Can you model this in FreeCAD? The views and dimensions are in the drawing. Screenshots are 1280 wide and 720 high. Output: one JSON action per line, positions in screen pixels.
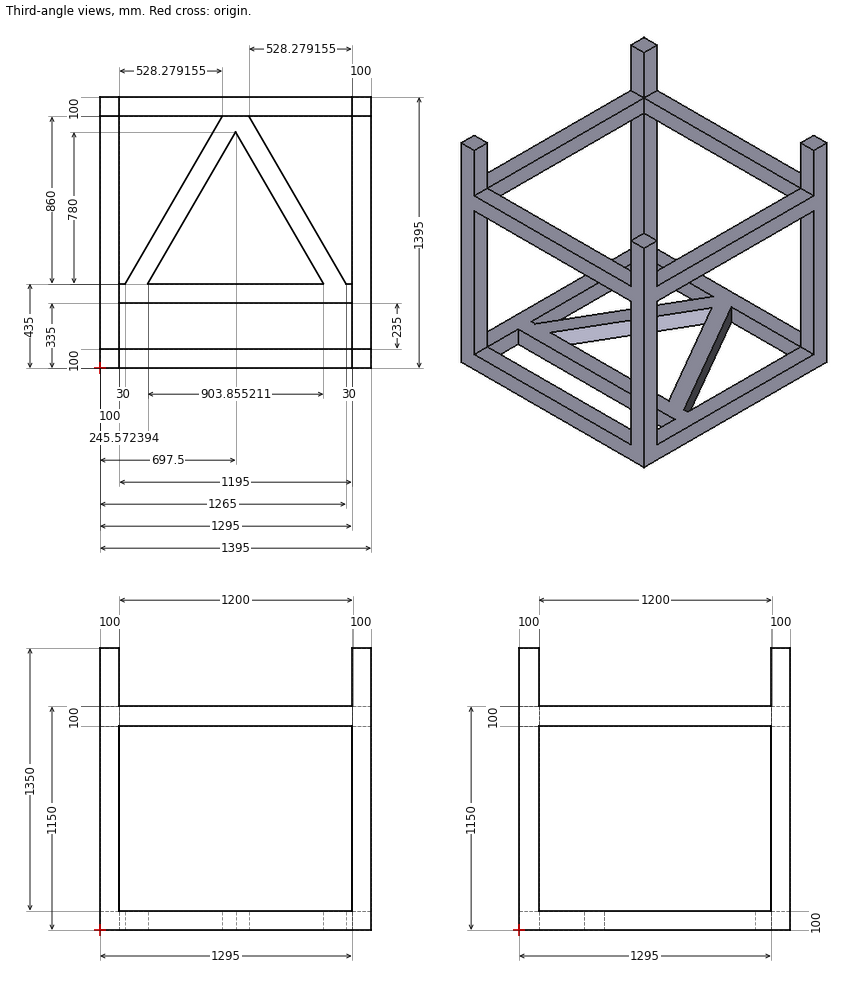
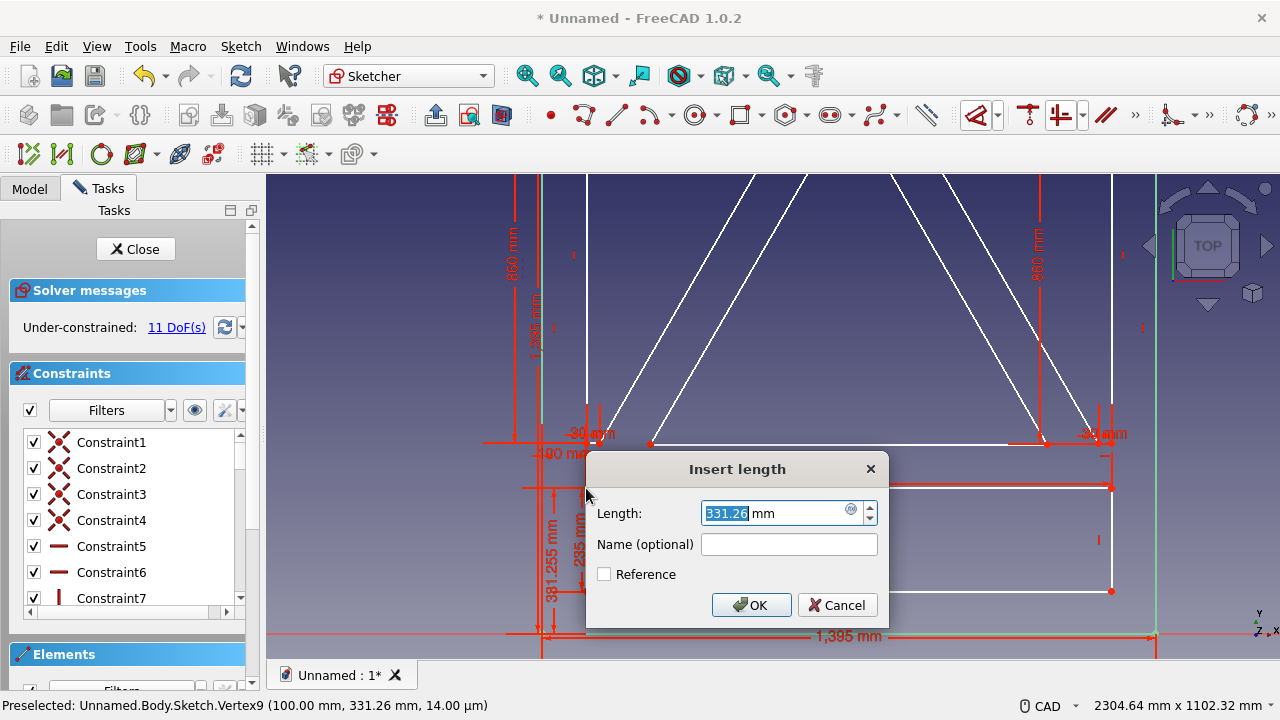
{"action": "type", "text": "335"}
{"action": "key", "text": "Return"}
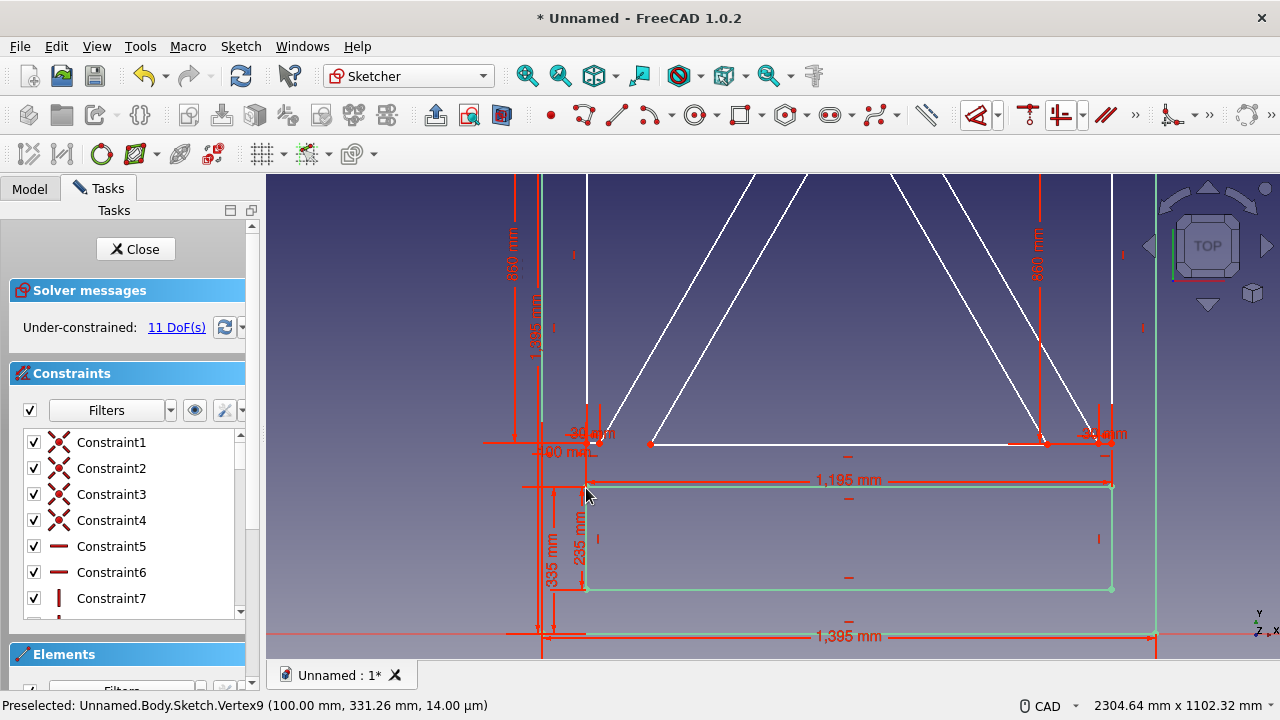
{"action": "left_click", "coordinate": [587, 443]}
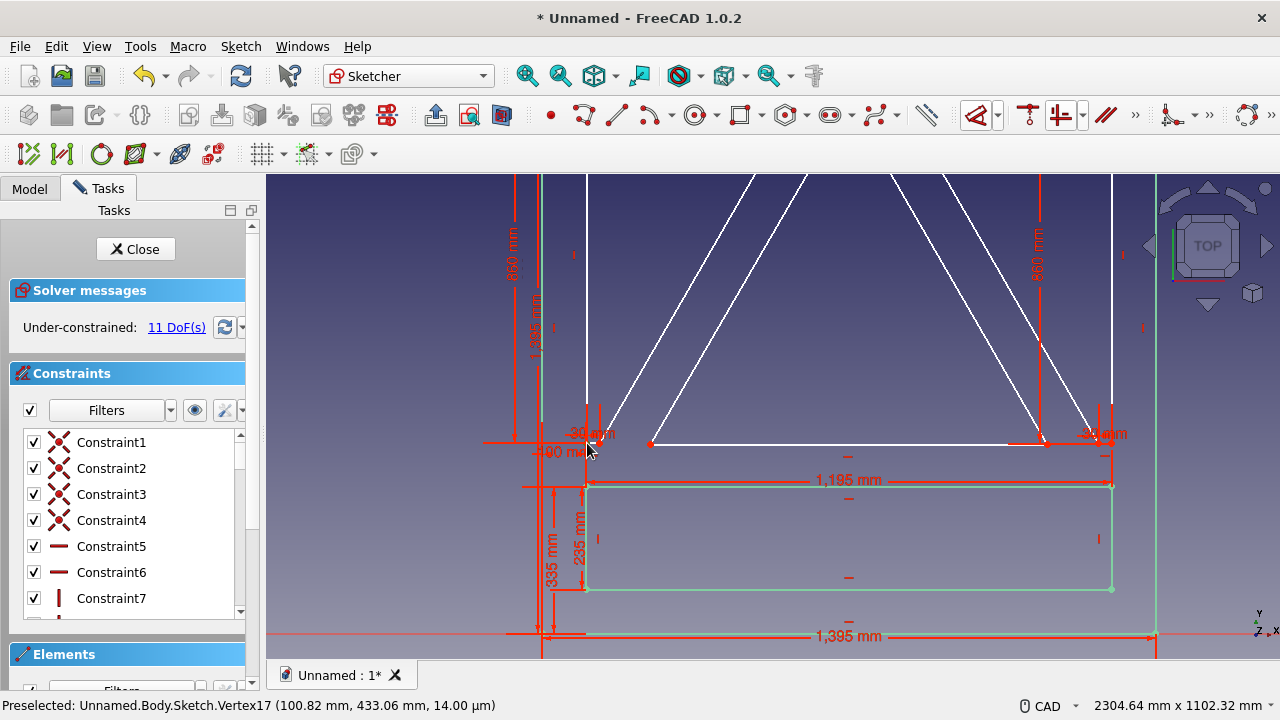
{"action": "left_click", "coordinate": [998, 116]}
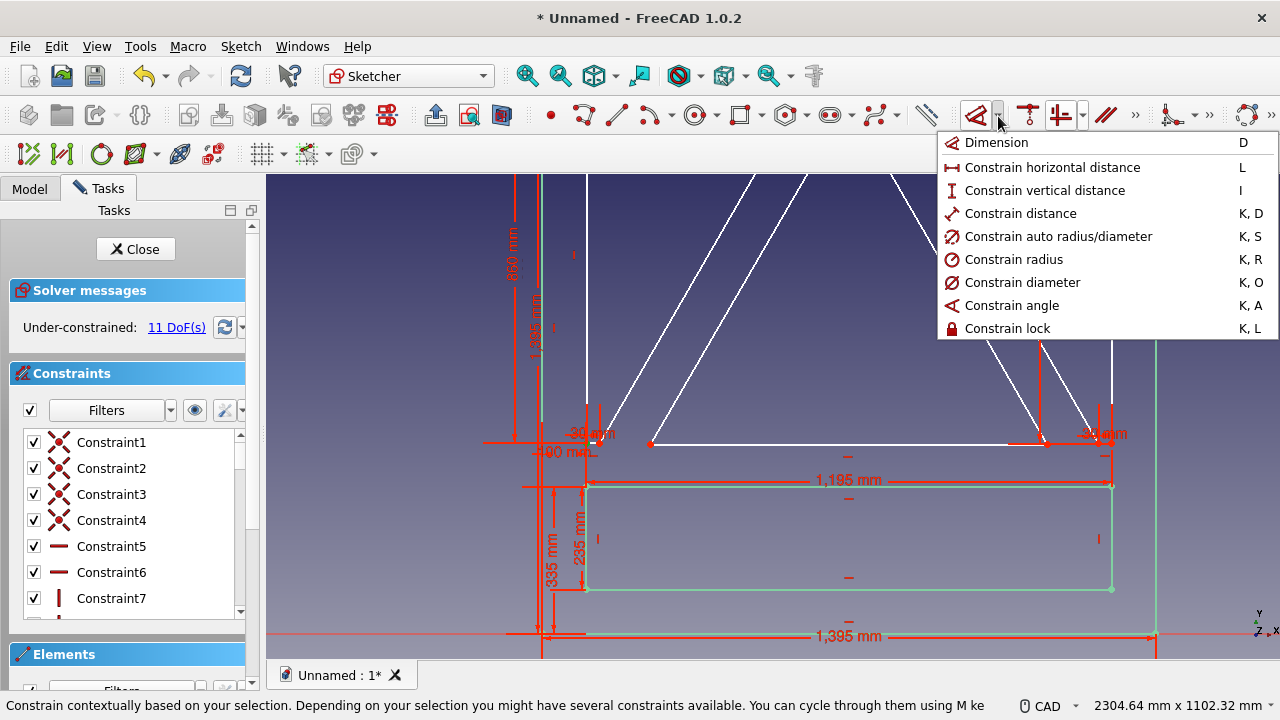
{"action": "left_click", "coordinate": [1108, 168]}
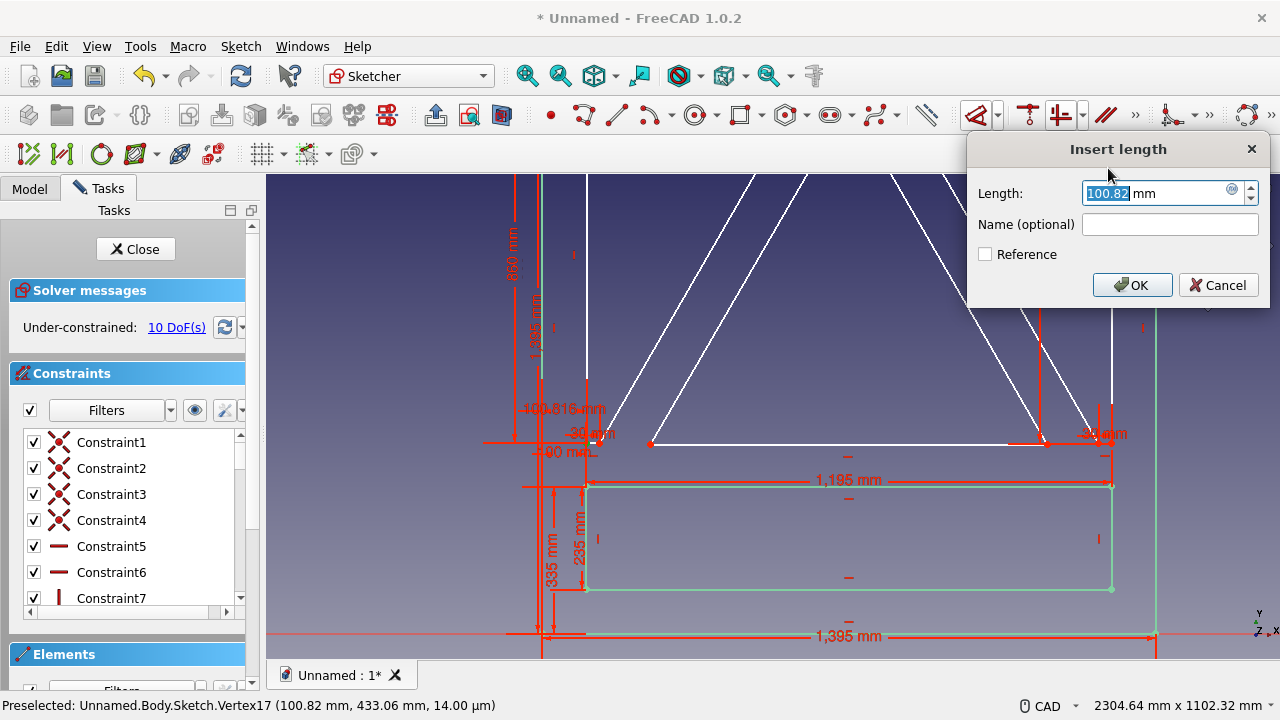
{"action": "type", "text": "100"}
{"action": "key", "text": "Return"}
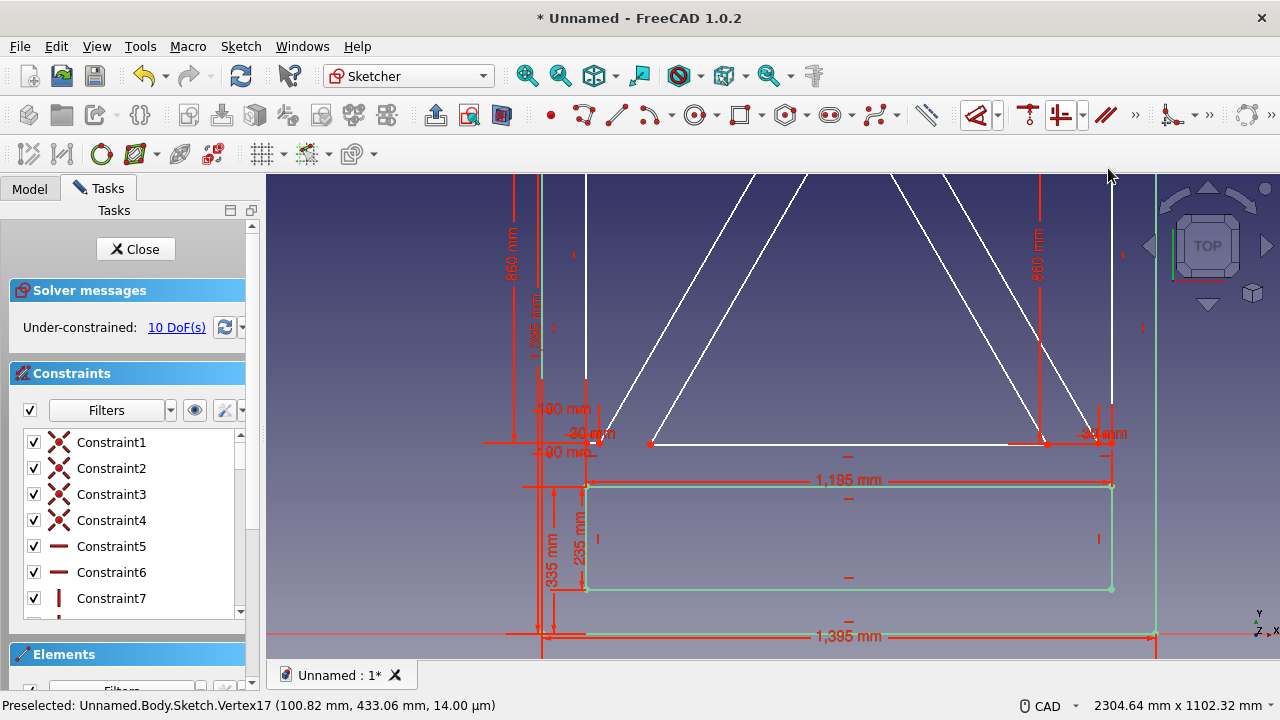
{"action": "left_click", "coordinate": [586, 443]}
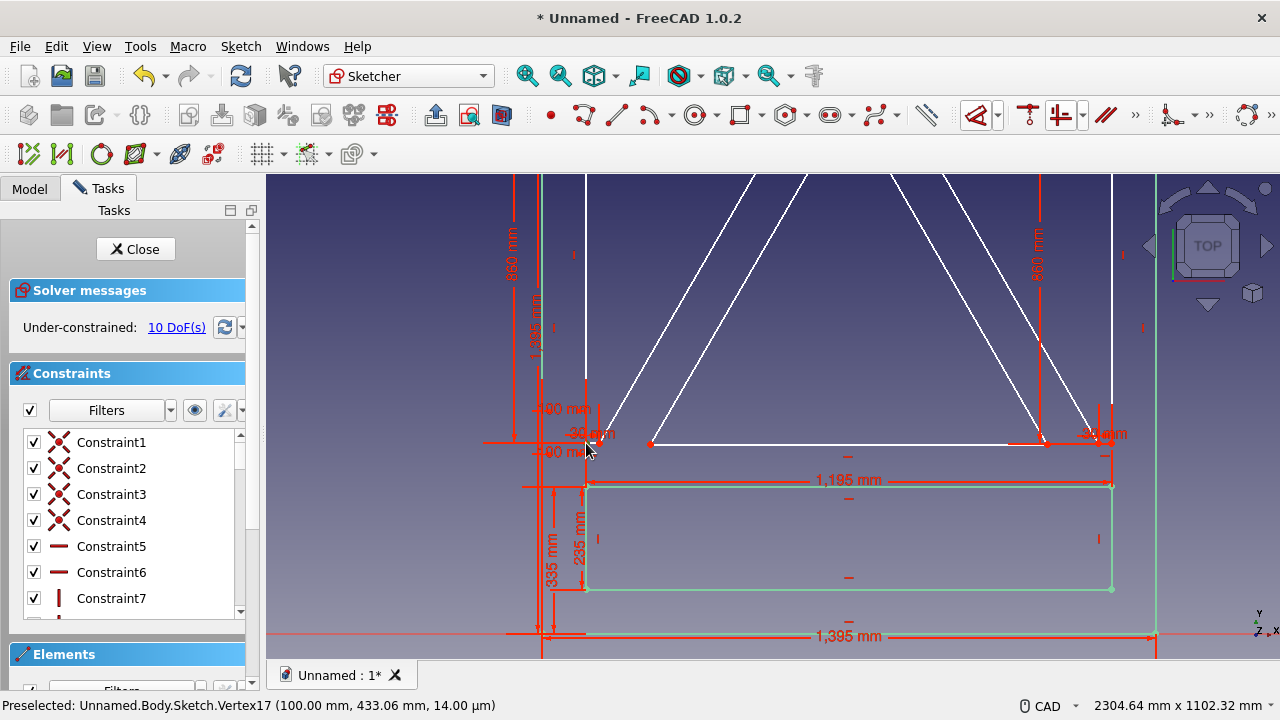
{"action": "key", "text": "i"}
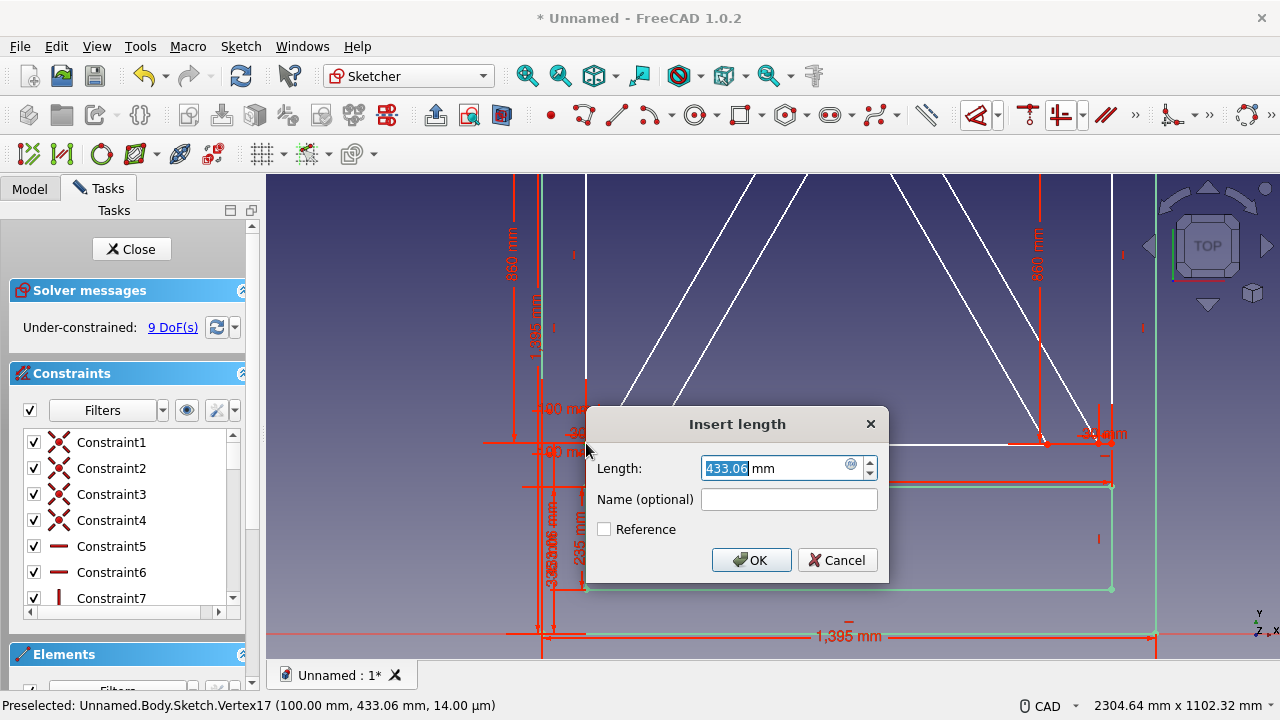
{"action": "type", "text": "435"}
{"action": "key", "text": "Return"}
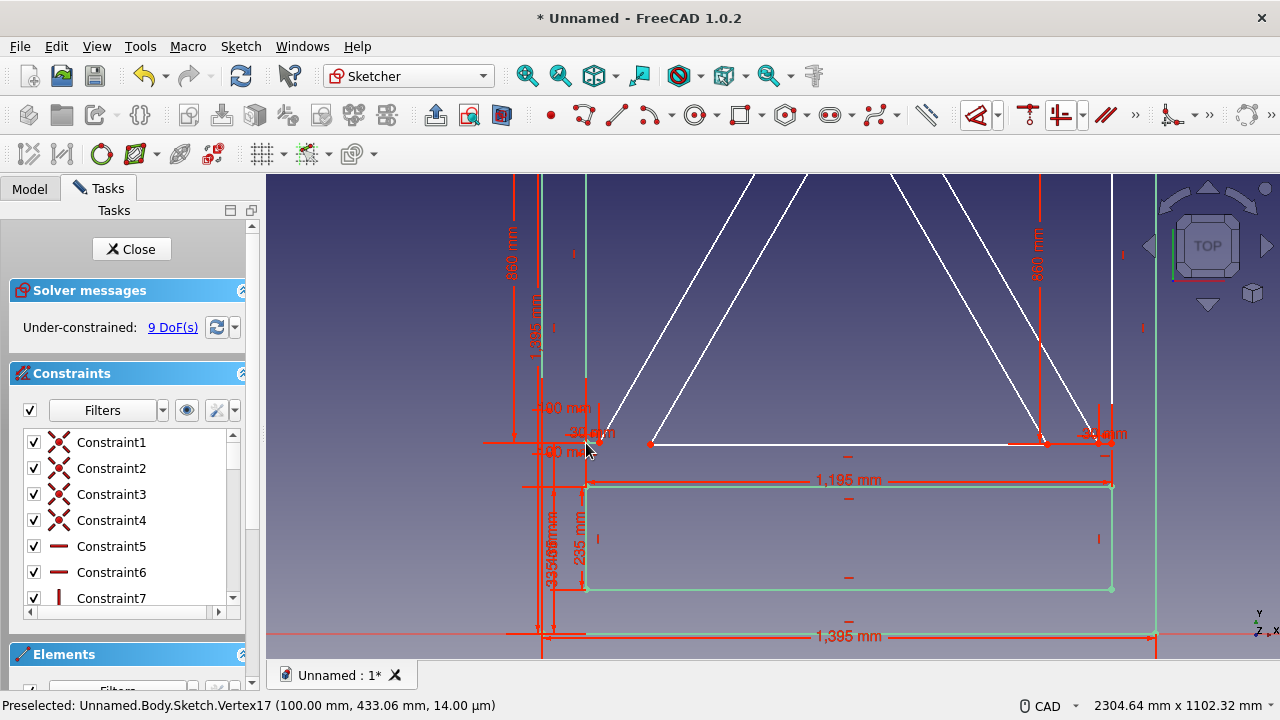
{"action": "left_click", "coordinate": [650, 445]}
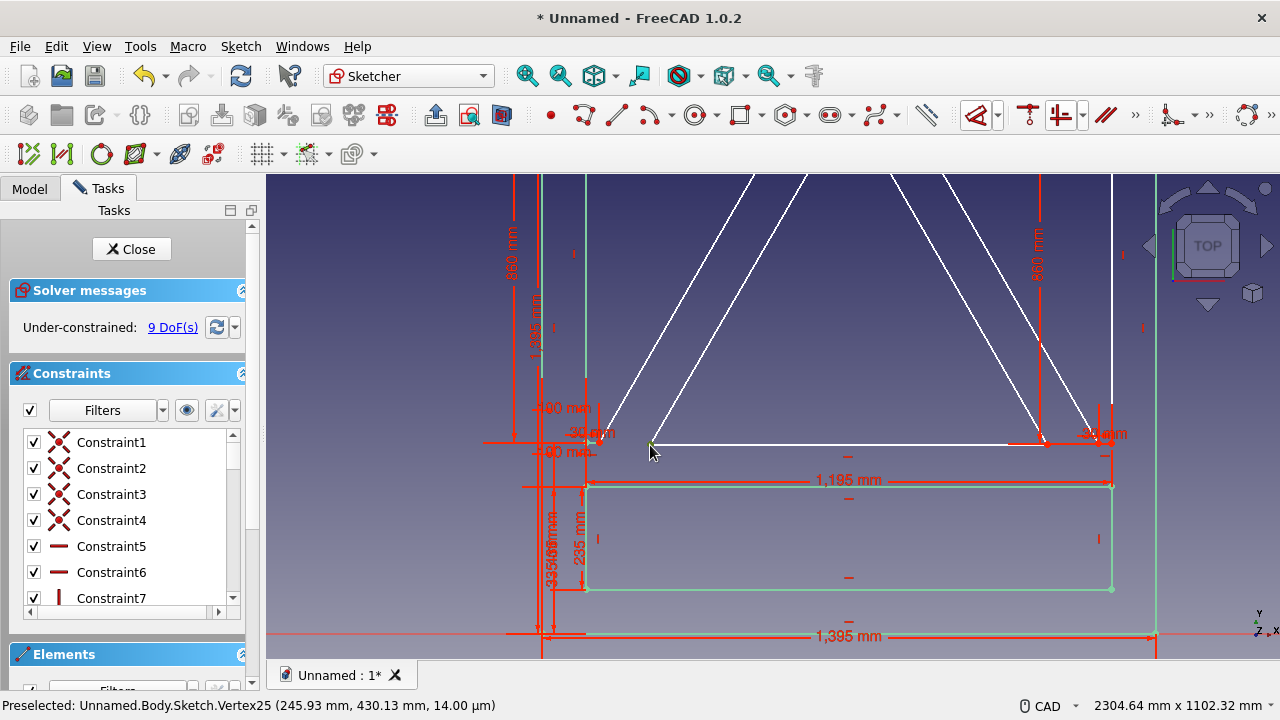
{"action": "left_click", "coordinate": [998, 116]}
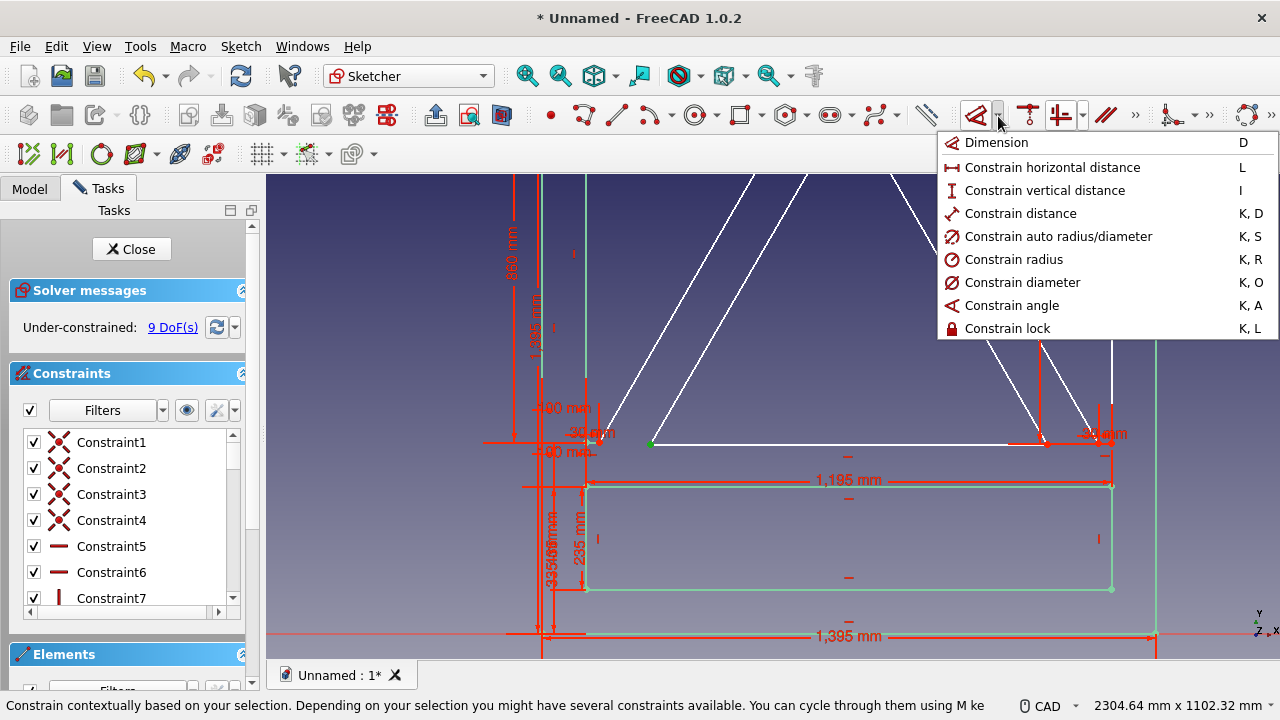
{"action": "left_click", "coordinate": [1108, 190]}